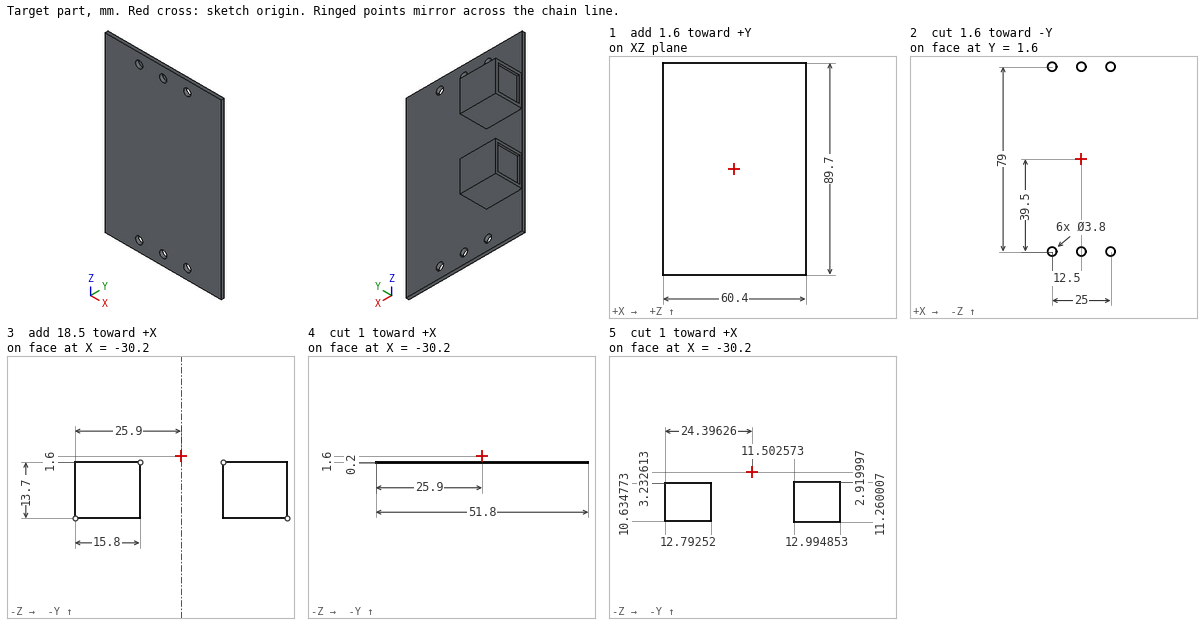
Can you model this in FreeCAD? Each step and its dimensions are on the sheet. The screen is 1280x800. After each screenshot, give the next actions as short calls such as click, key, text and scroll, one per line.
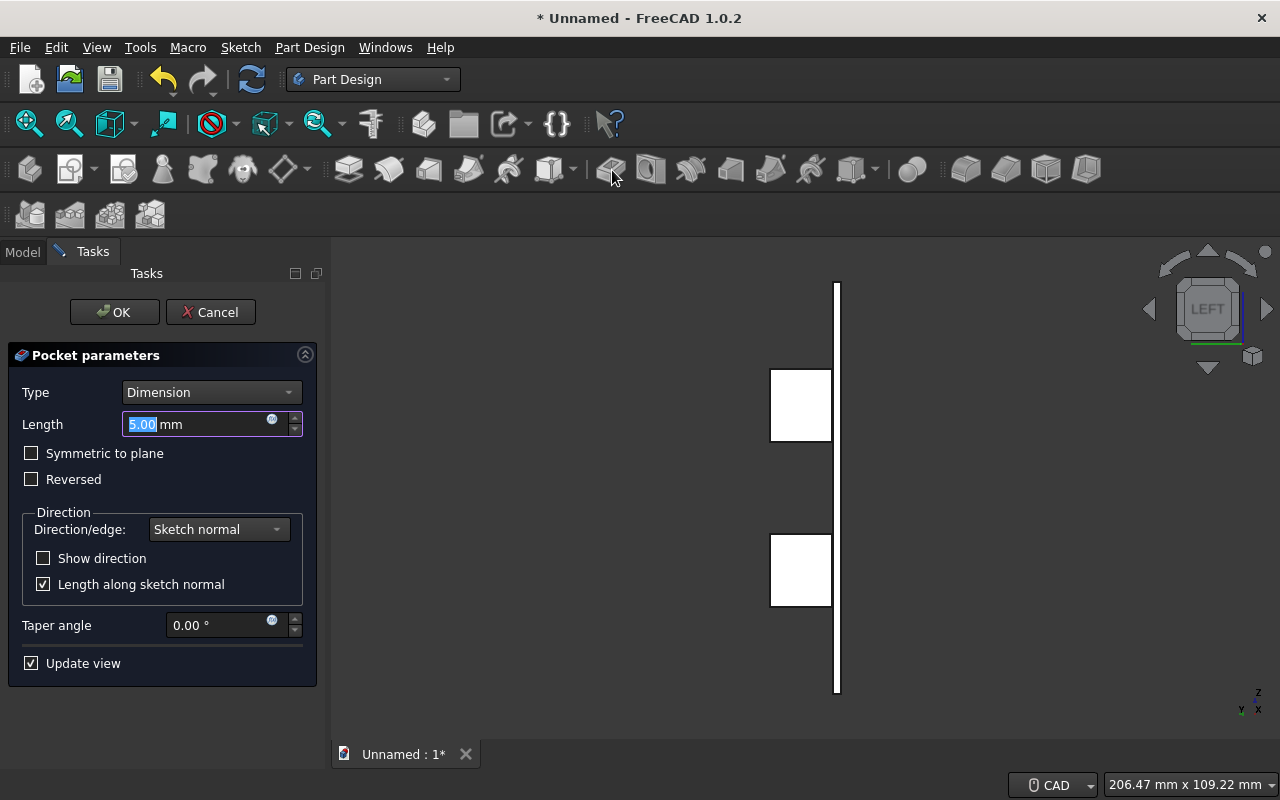
text(1)
key(Tab)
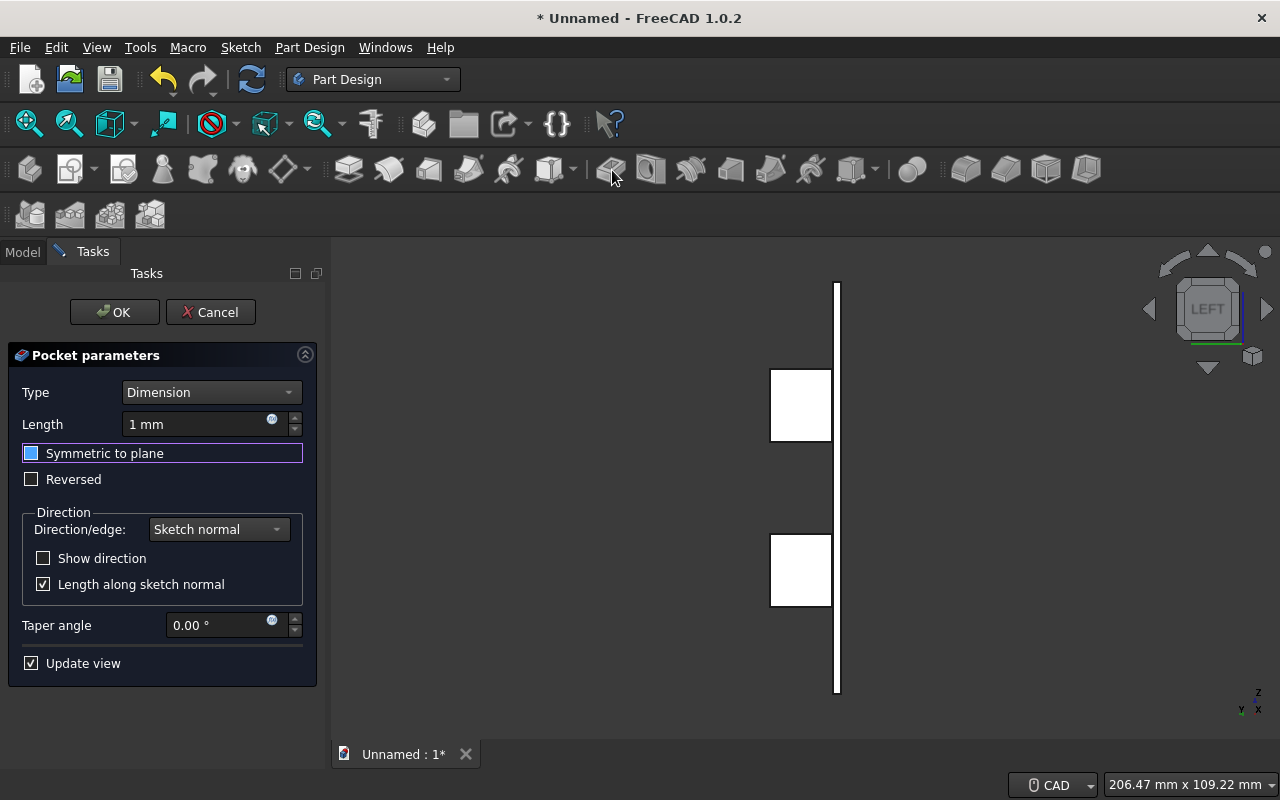
click(115, 312)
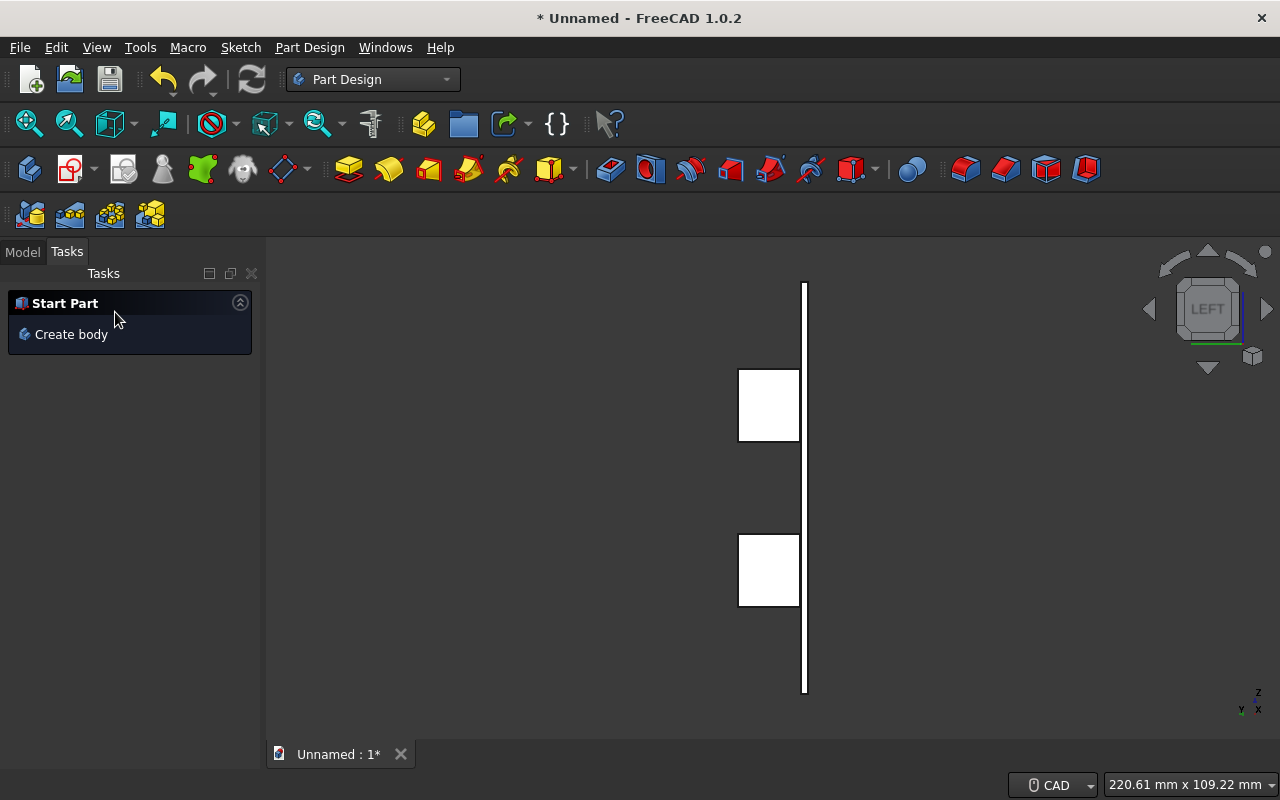
click(769, 570)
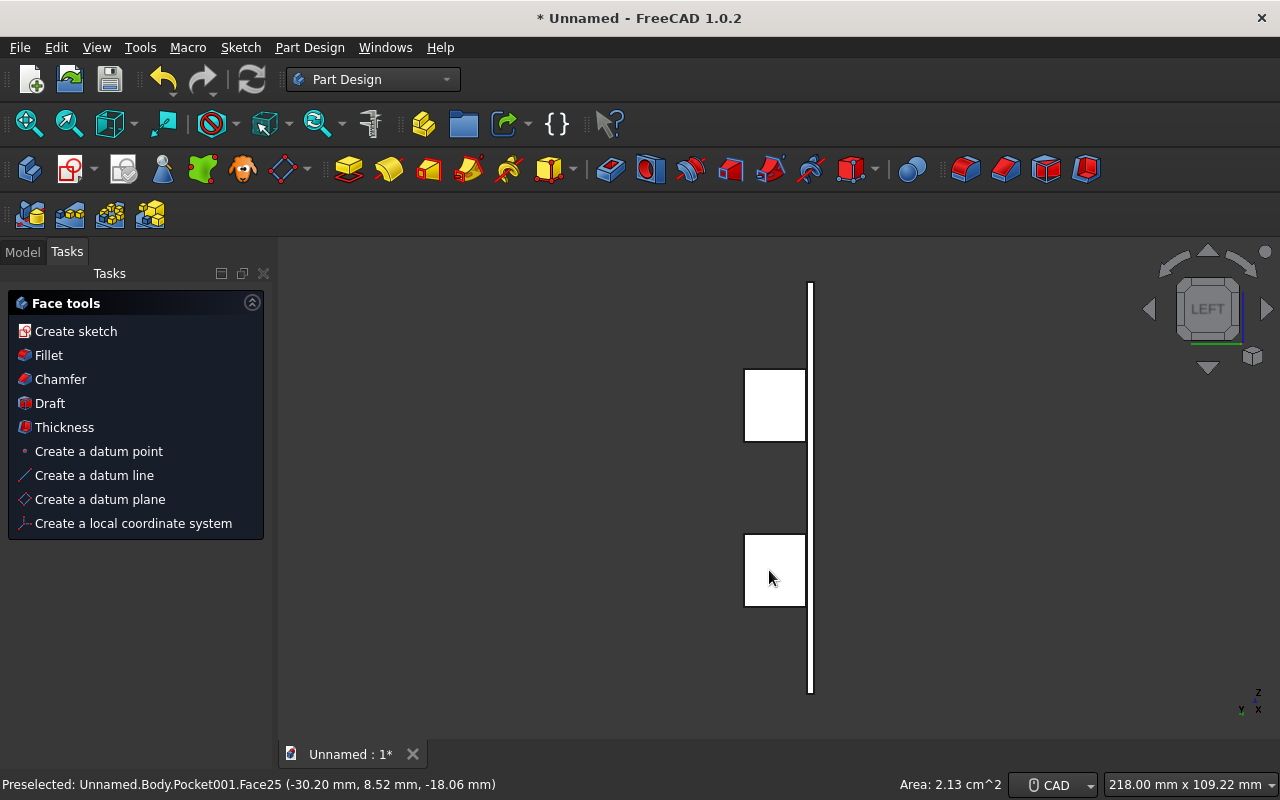
click(70, 170)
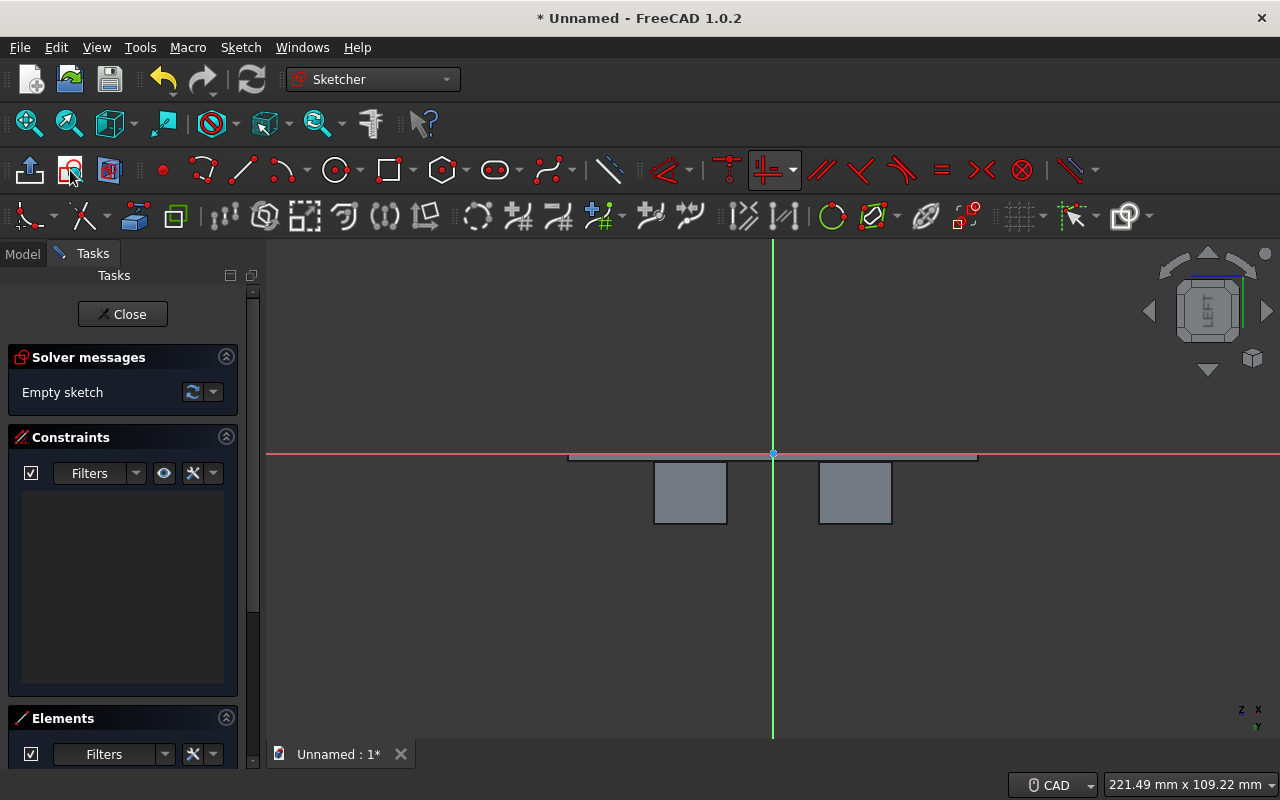
scroll(813, 485, up, 5)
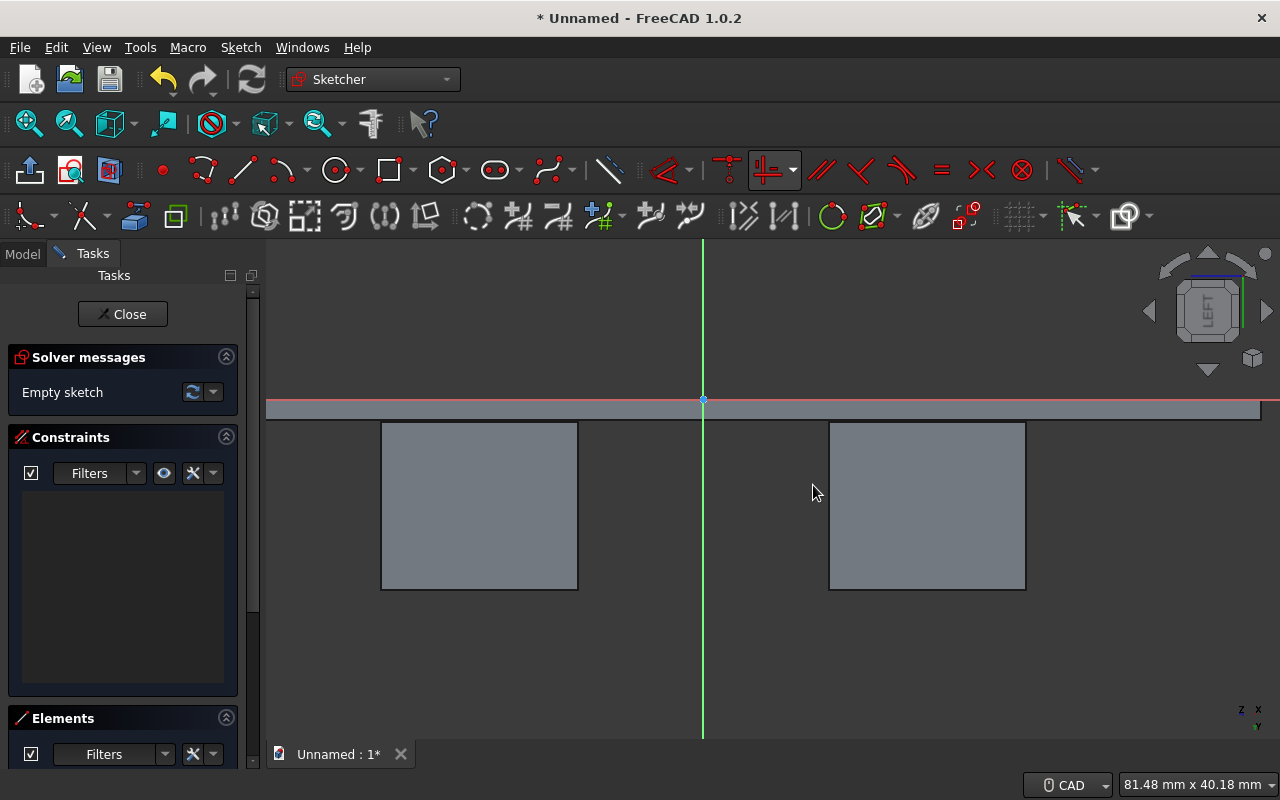
click(390, 170)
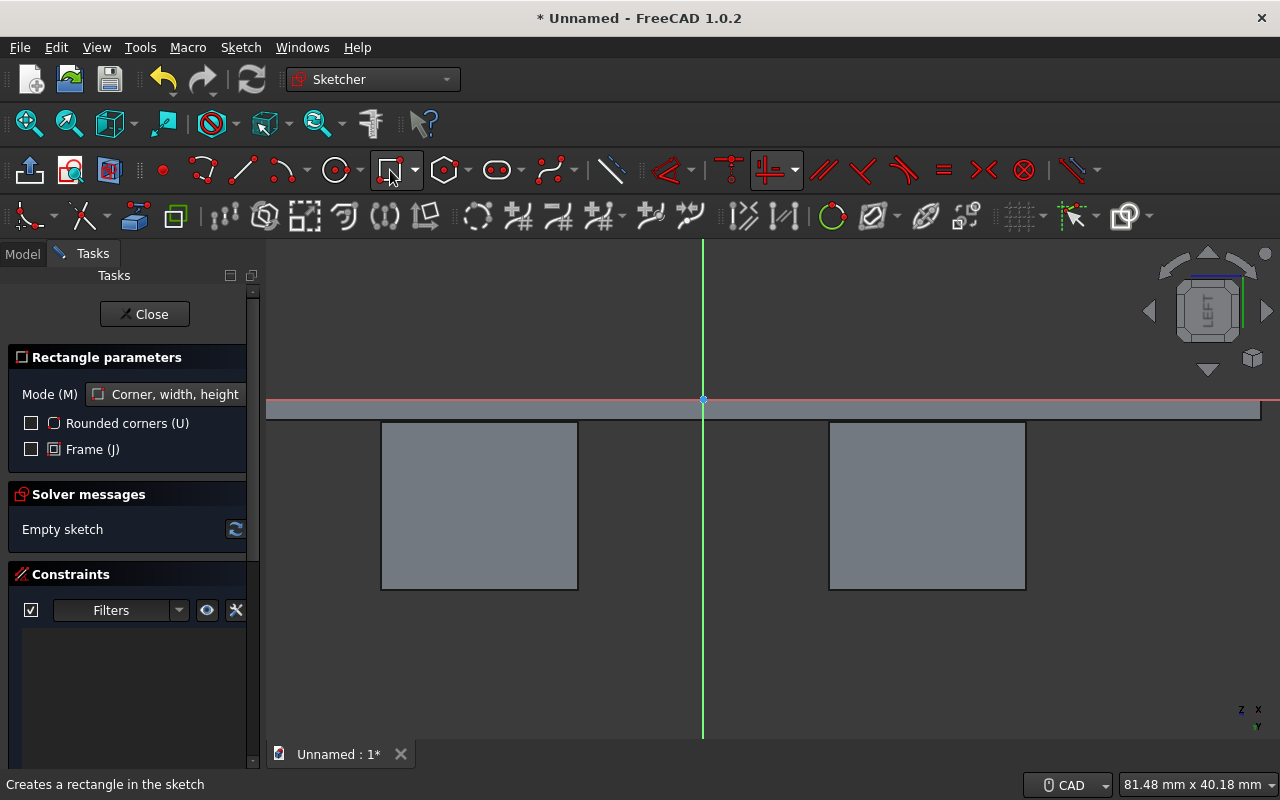
click(400, 440)
click(559, 572)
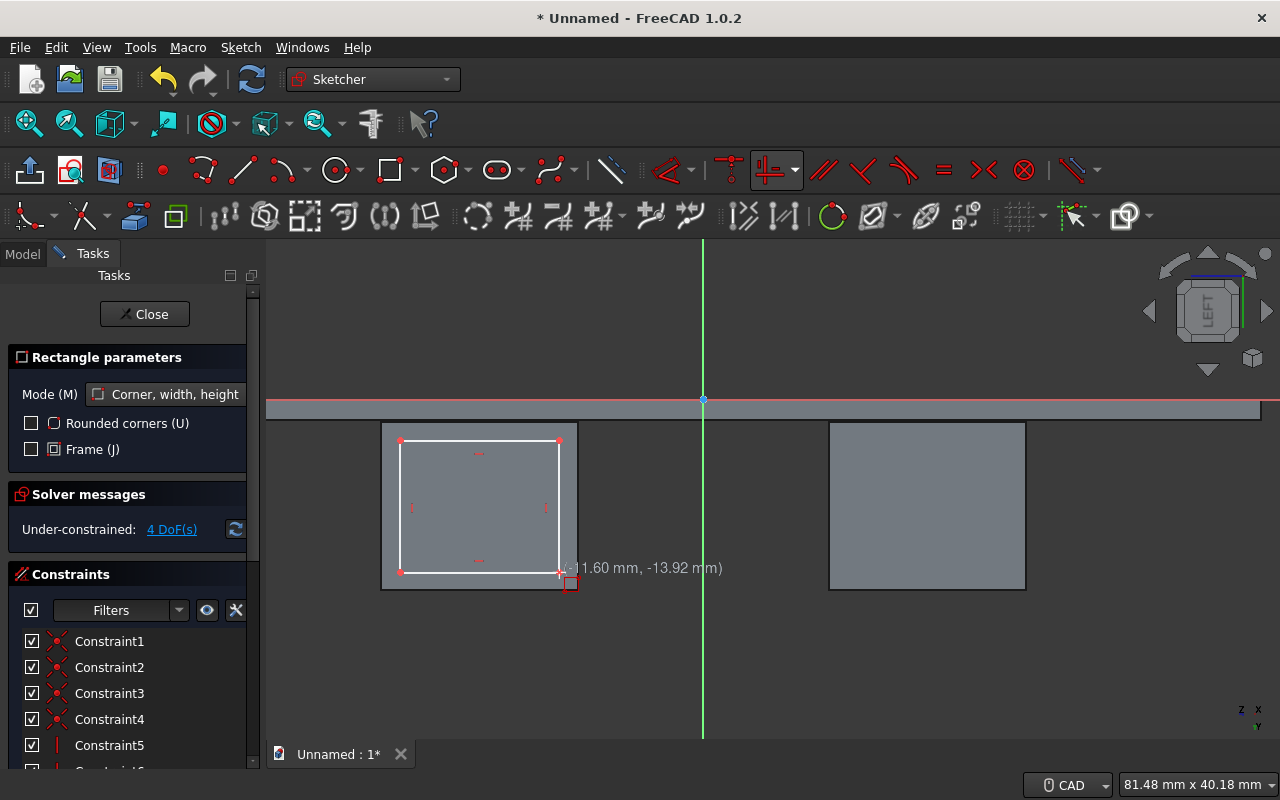
click(846, 436)
click(1008, 576)
key(Escape)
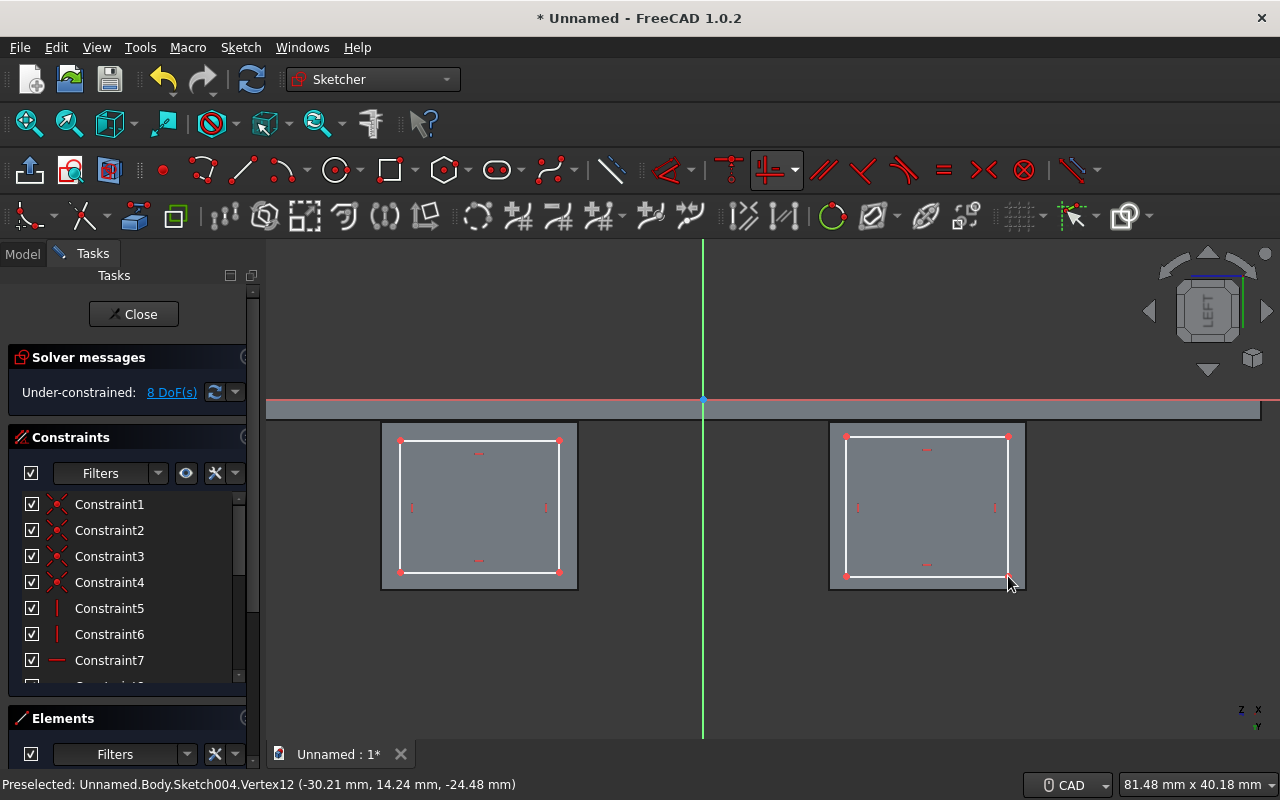
key(d)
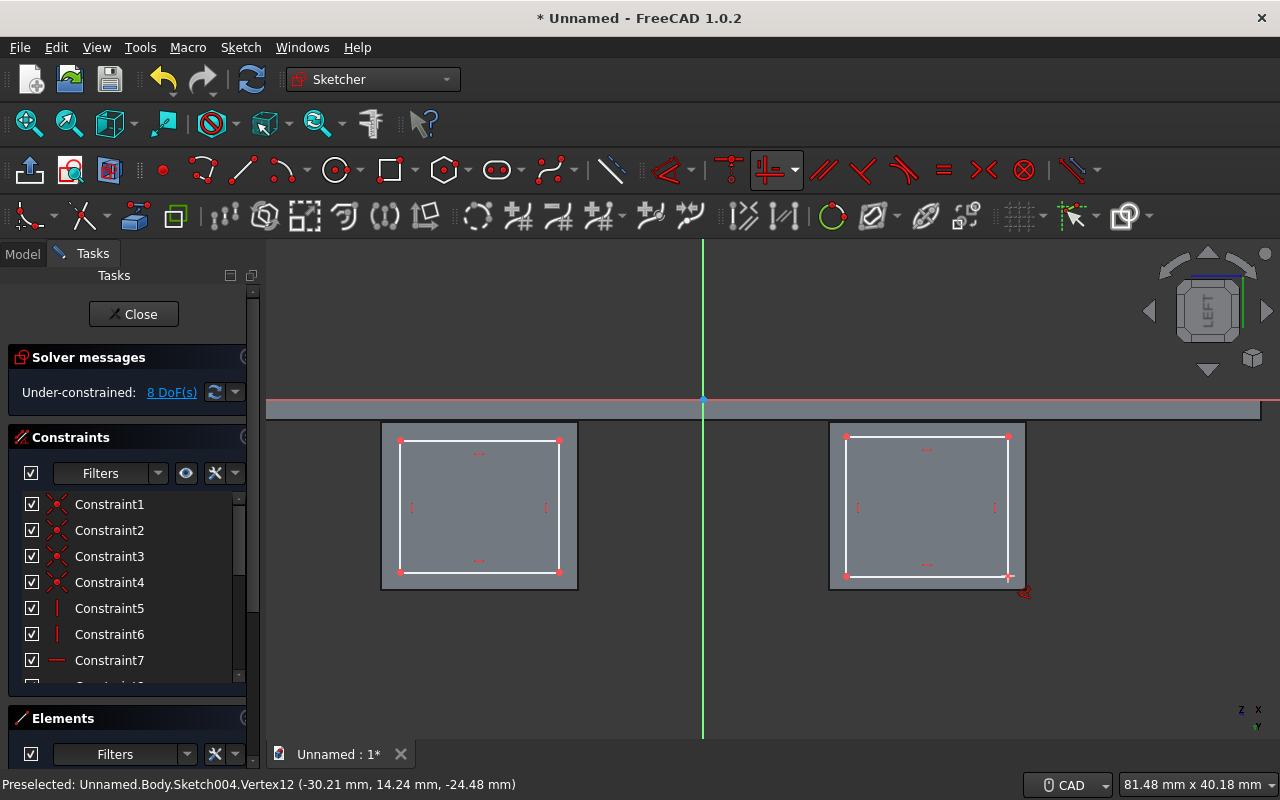
click(448, 573)
click(479, 607)